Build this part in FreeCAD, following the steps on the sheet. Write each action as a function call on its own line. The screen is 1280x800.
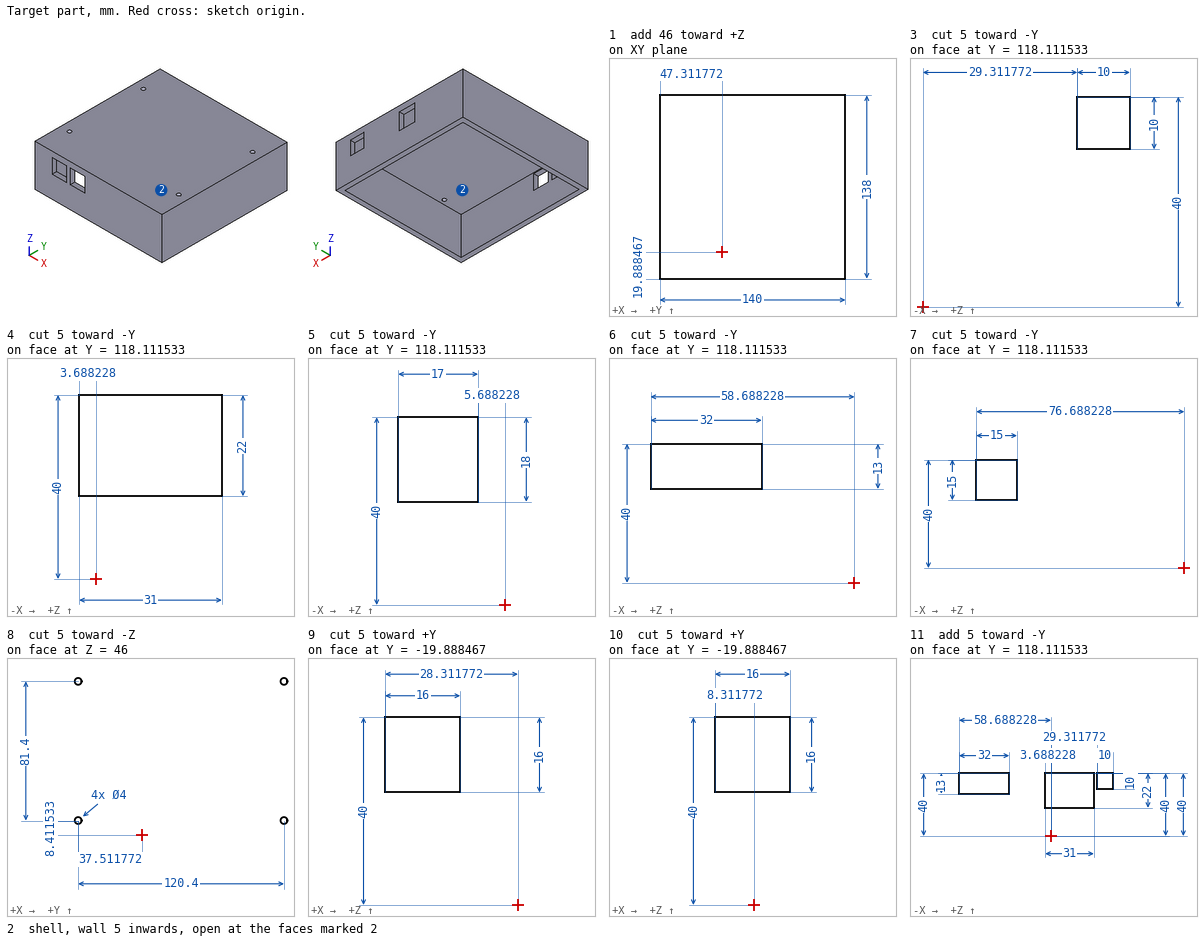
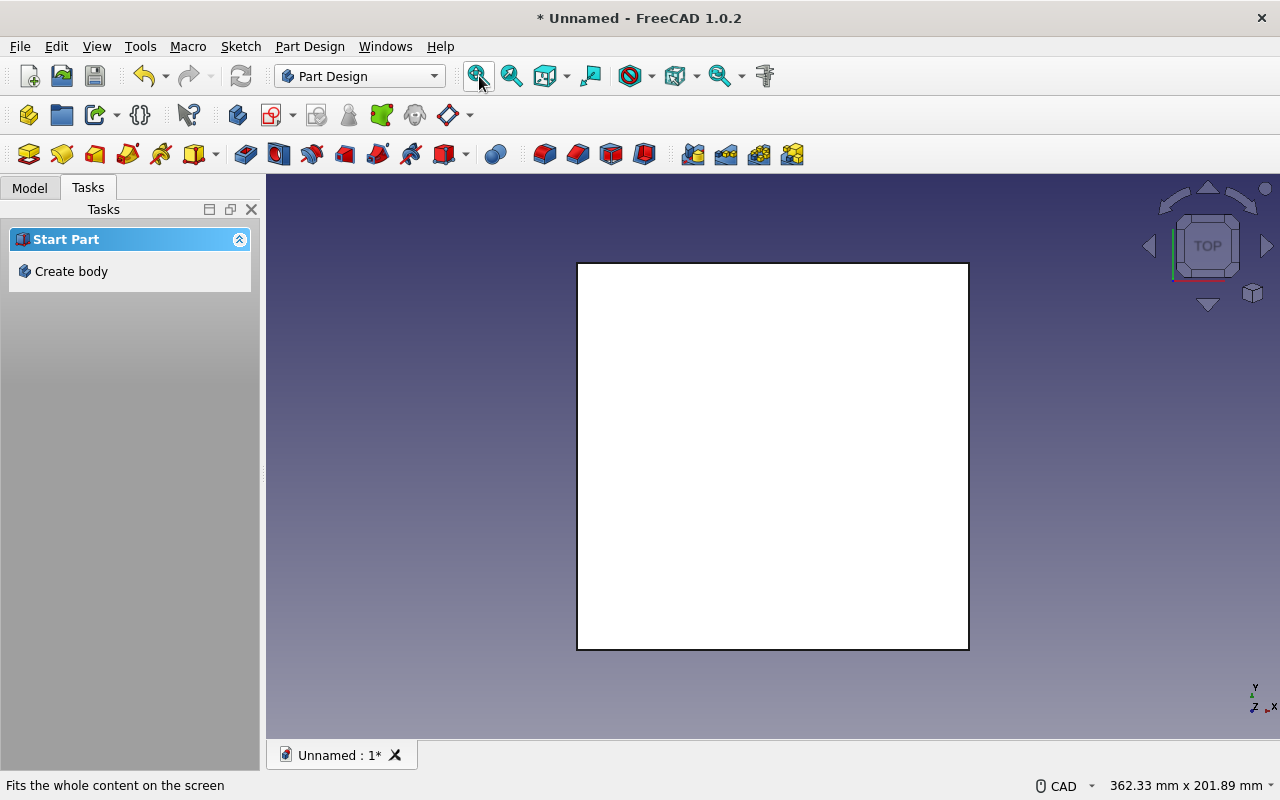
key(1)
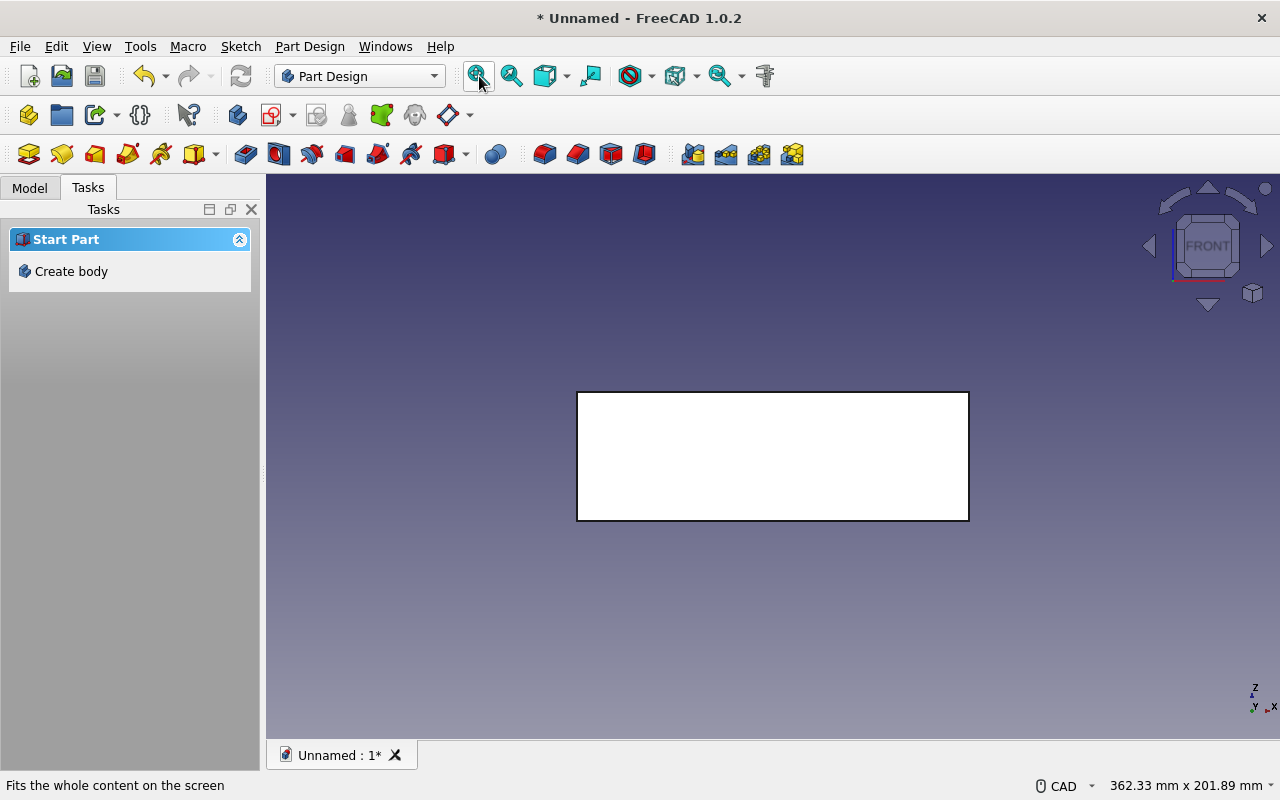
click(479, 76)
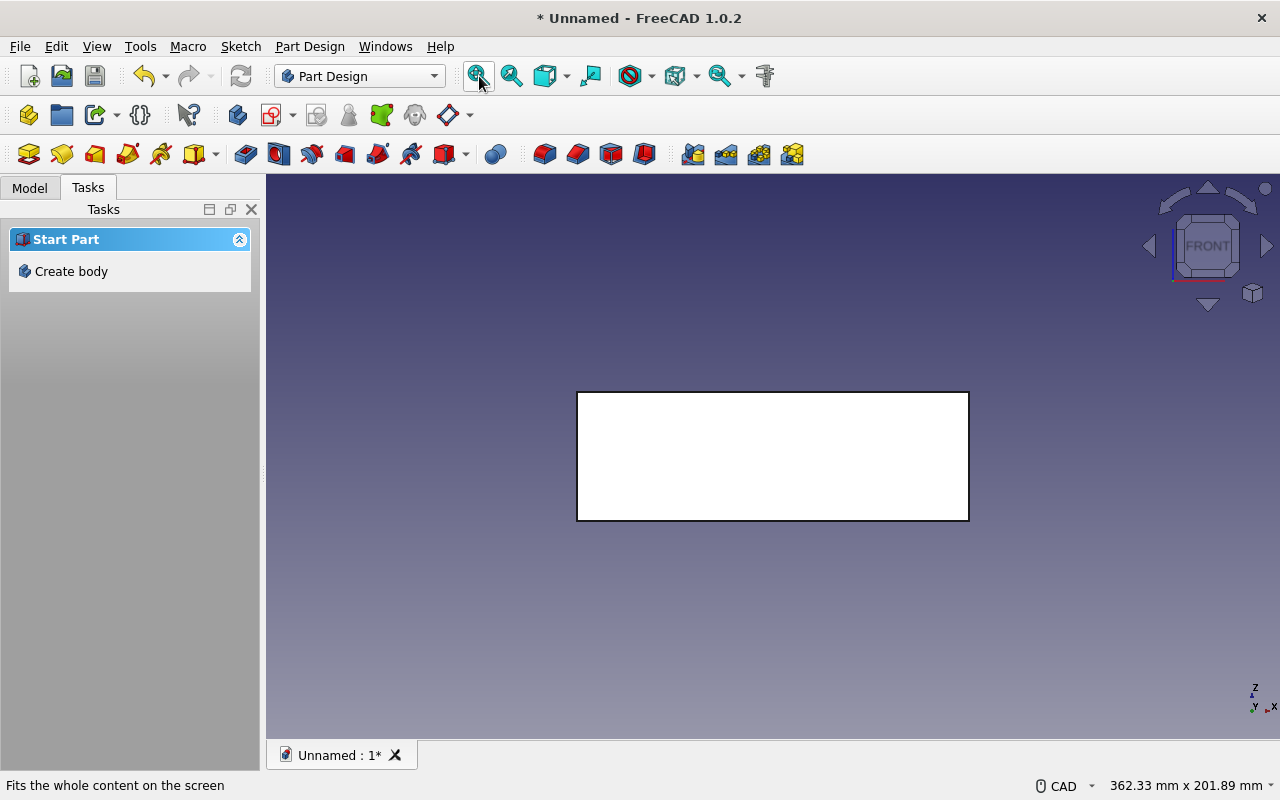
key(3)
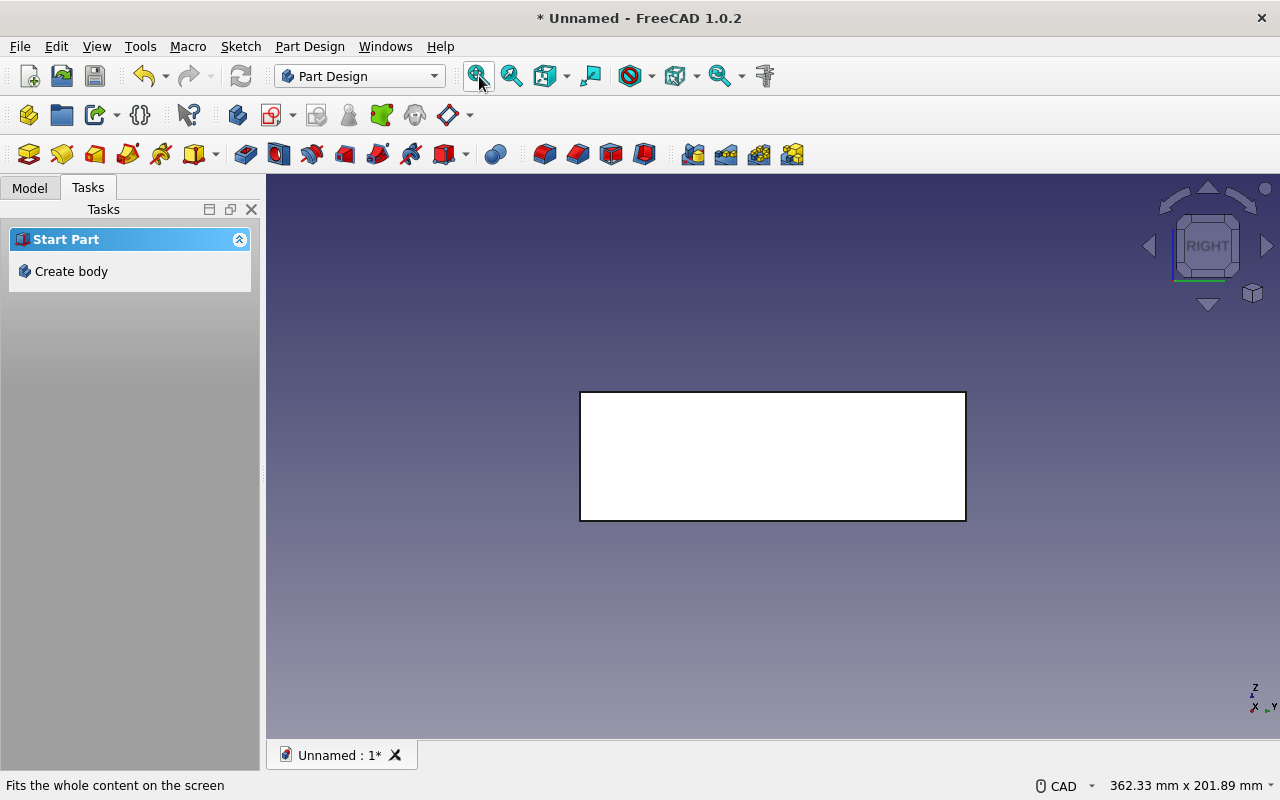
click(479, 76)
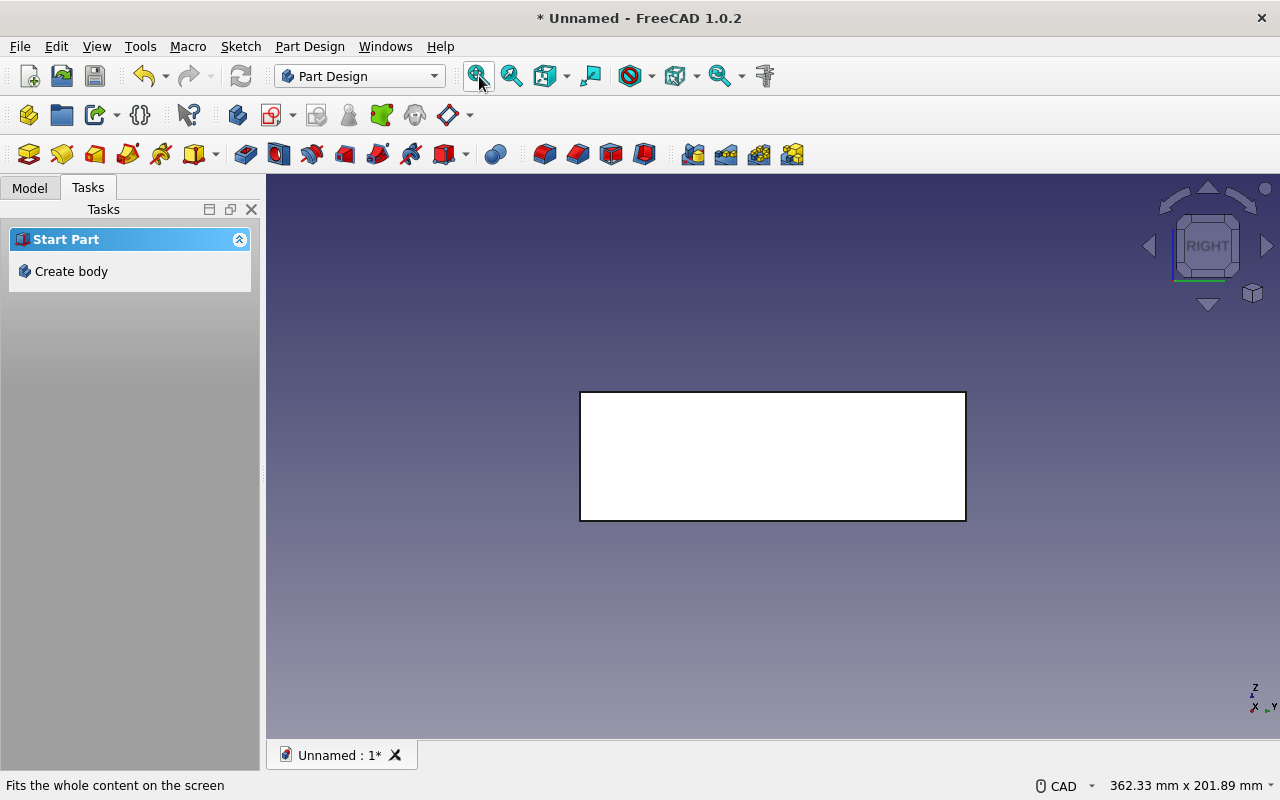
key(5)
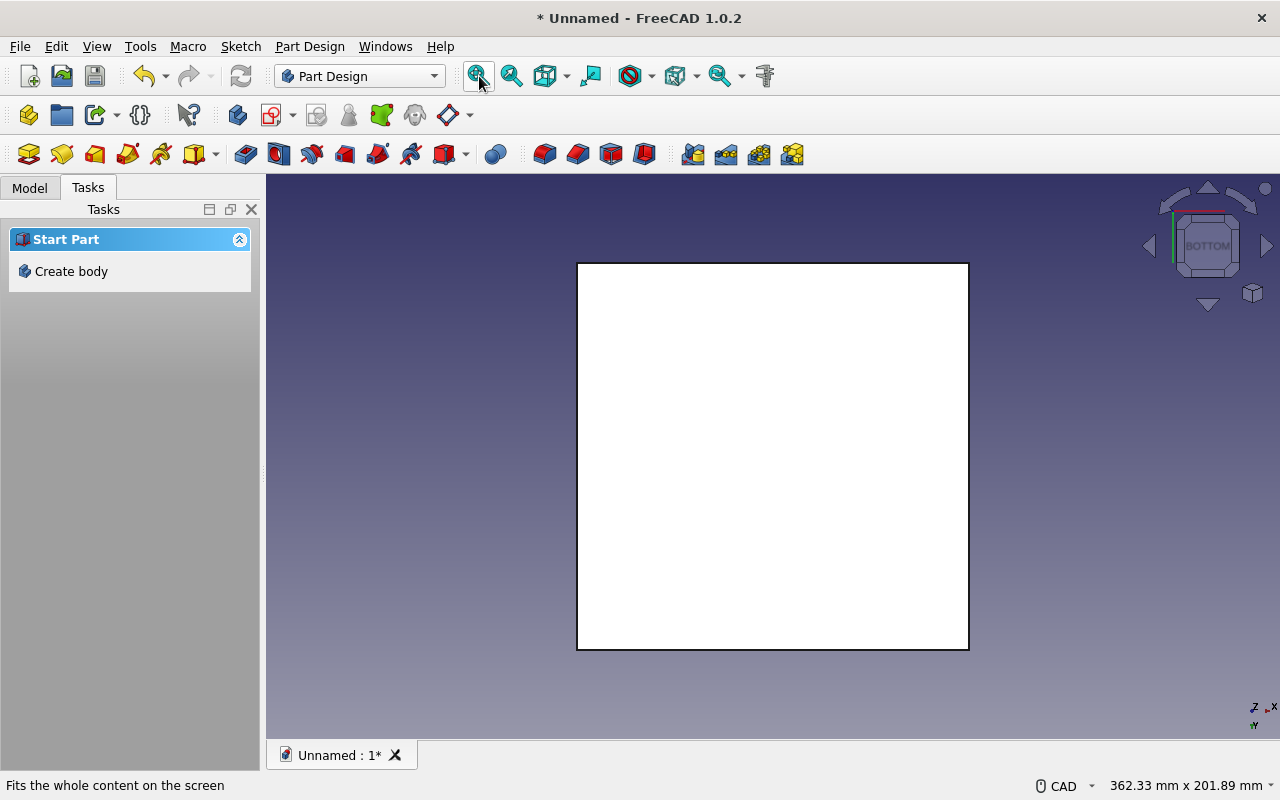
click(773, 455)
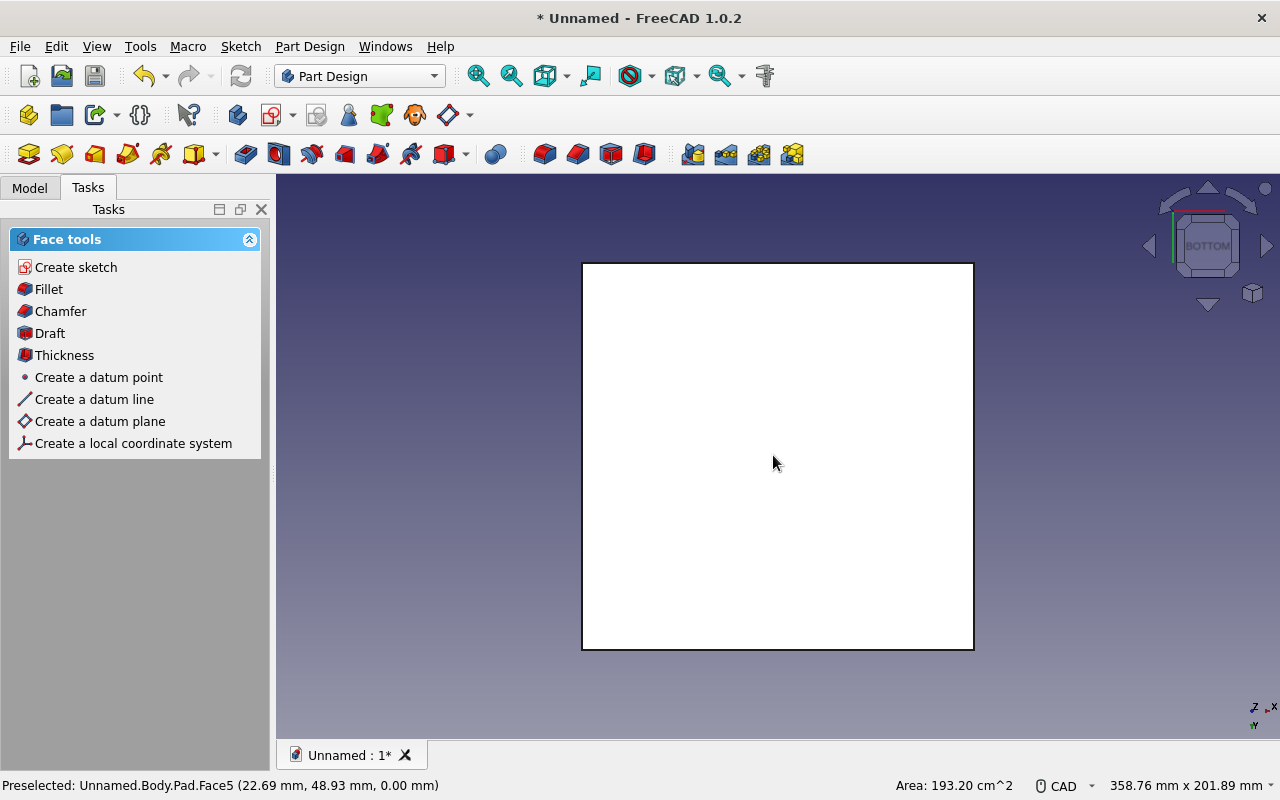
click(644, 154)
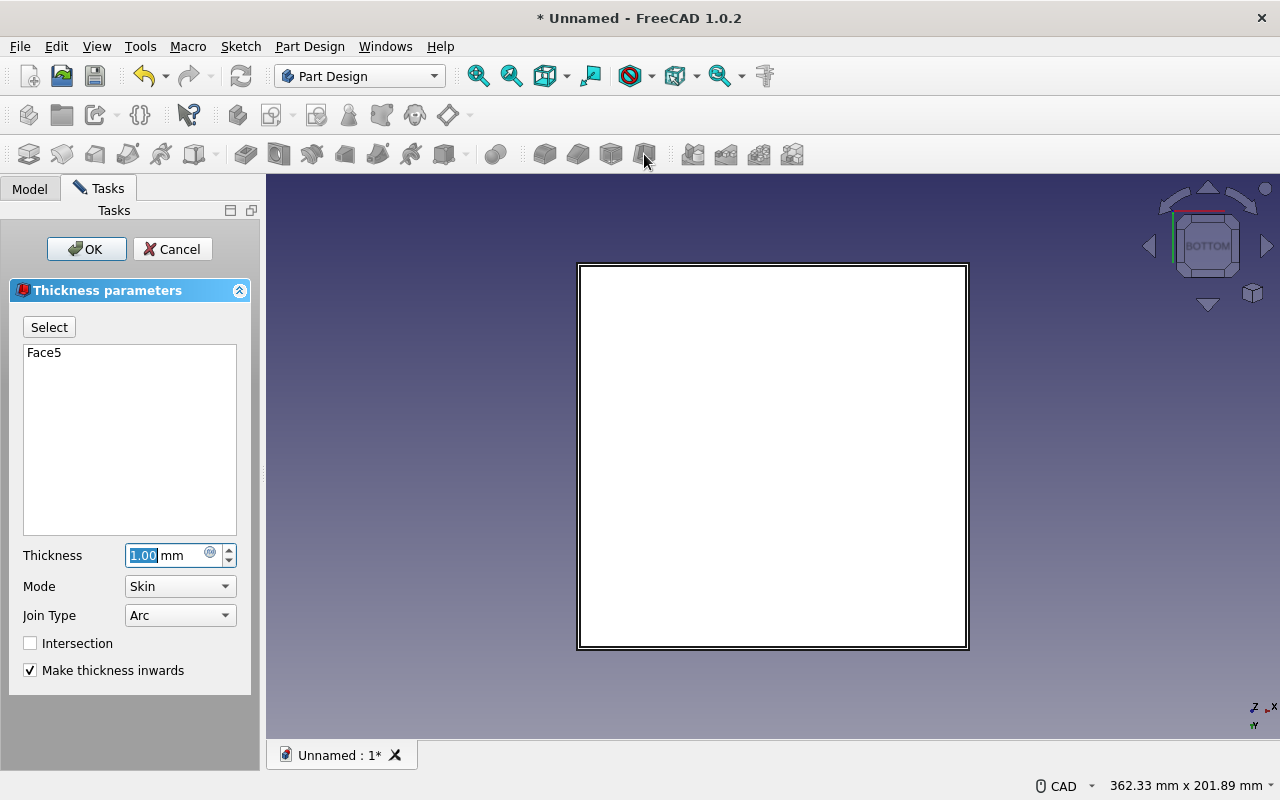
text(5)
key(Tab)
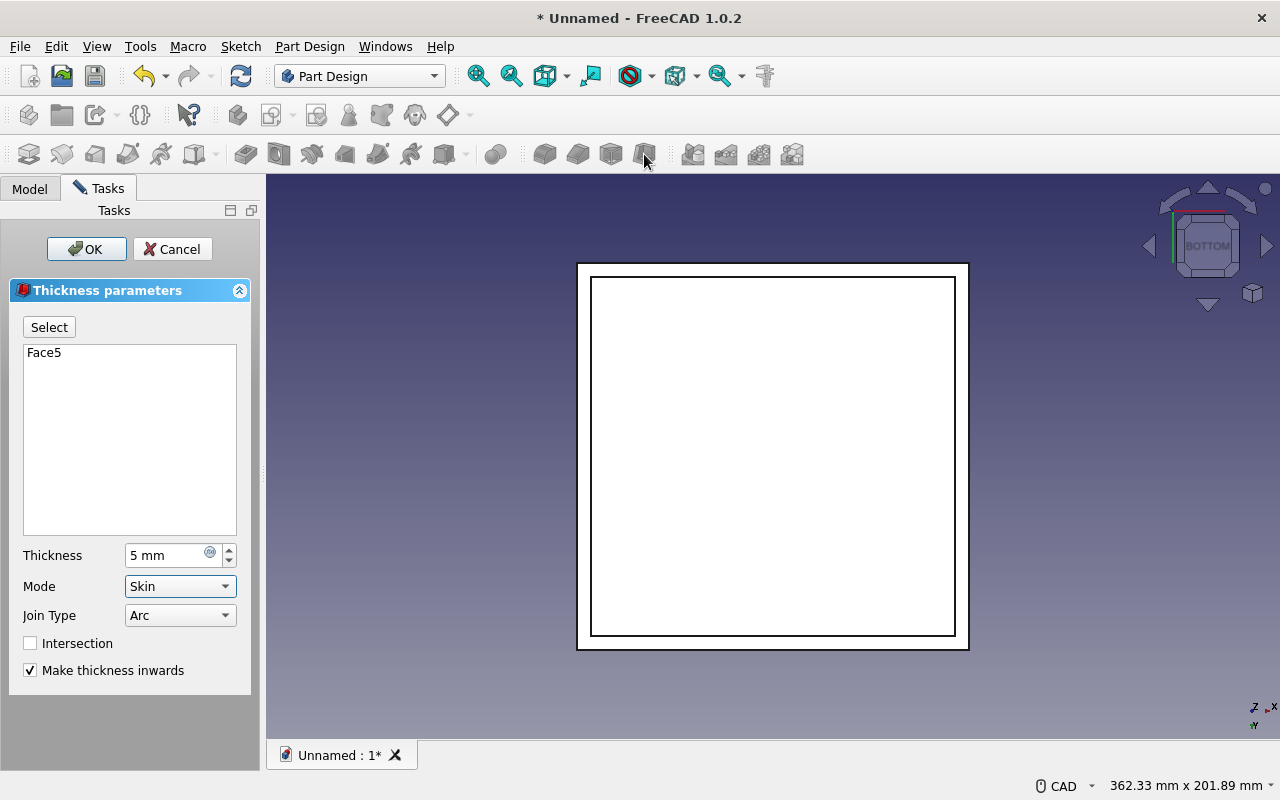
click(181, 616)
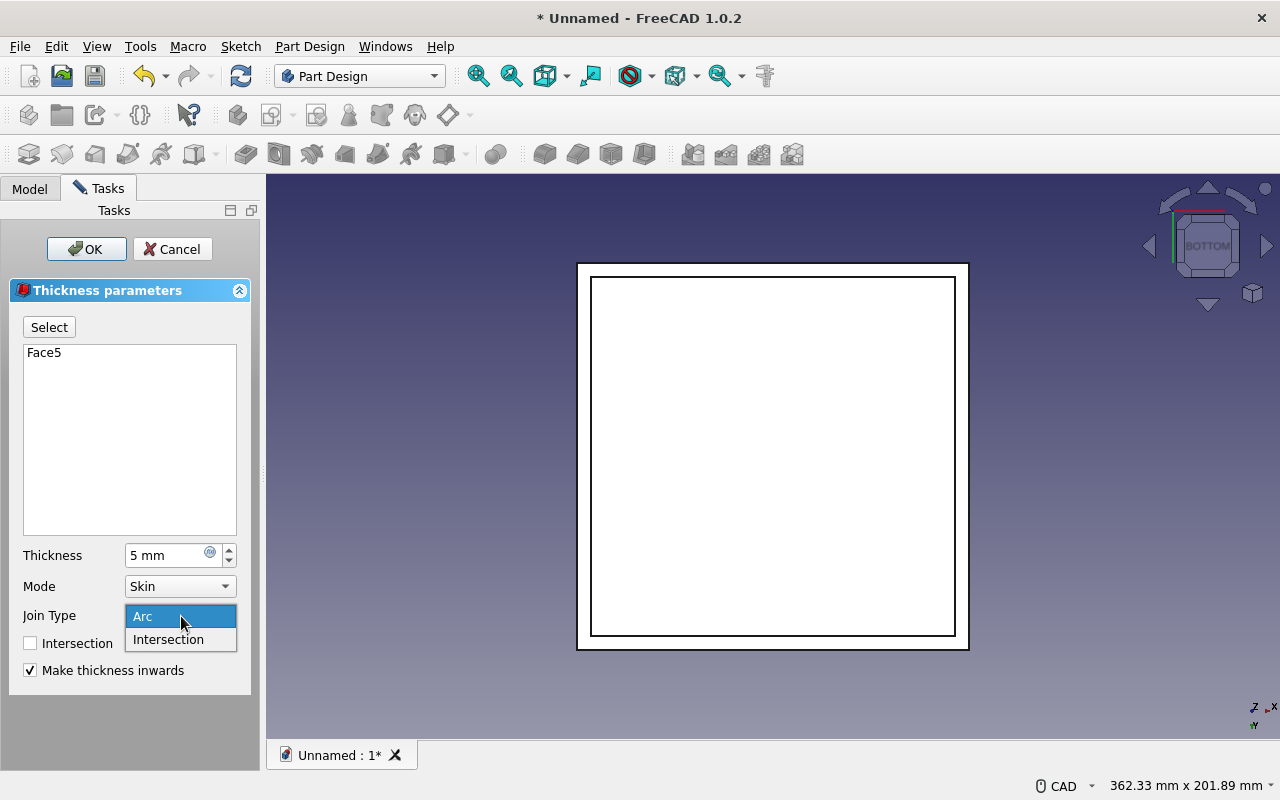
click(179, 640)